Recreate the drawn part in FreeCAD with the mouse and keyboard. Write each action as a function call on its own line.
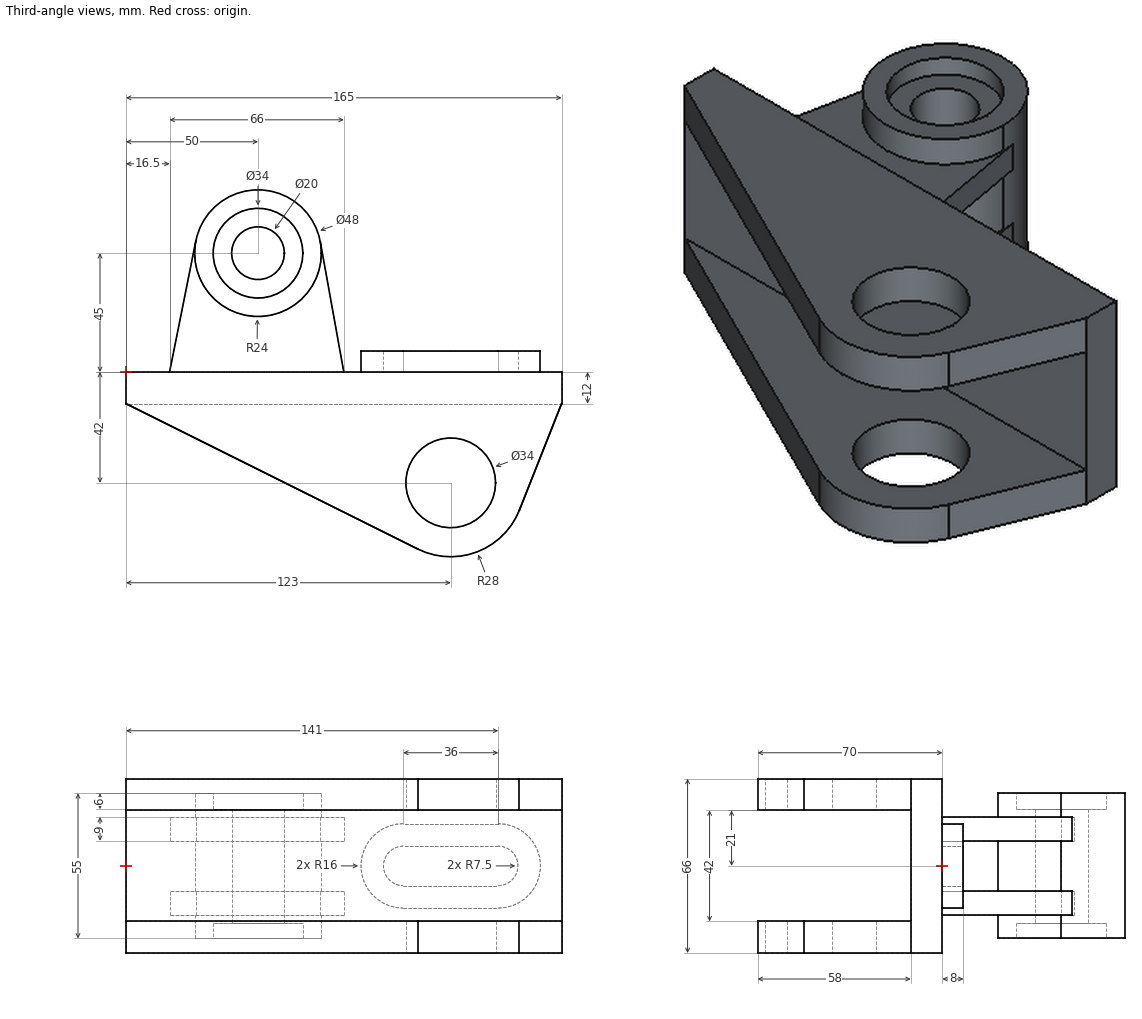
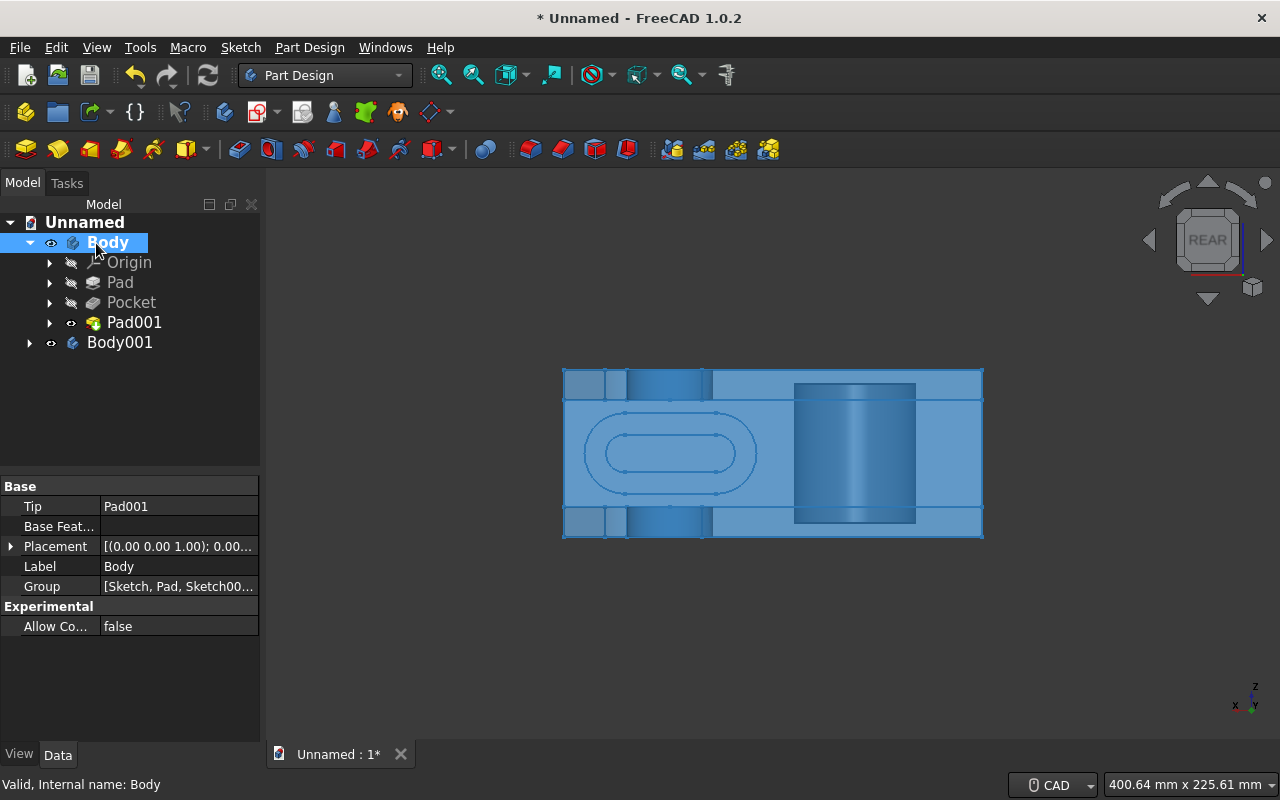
click(96, 243)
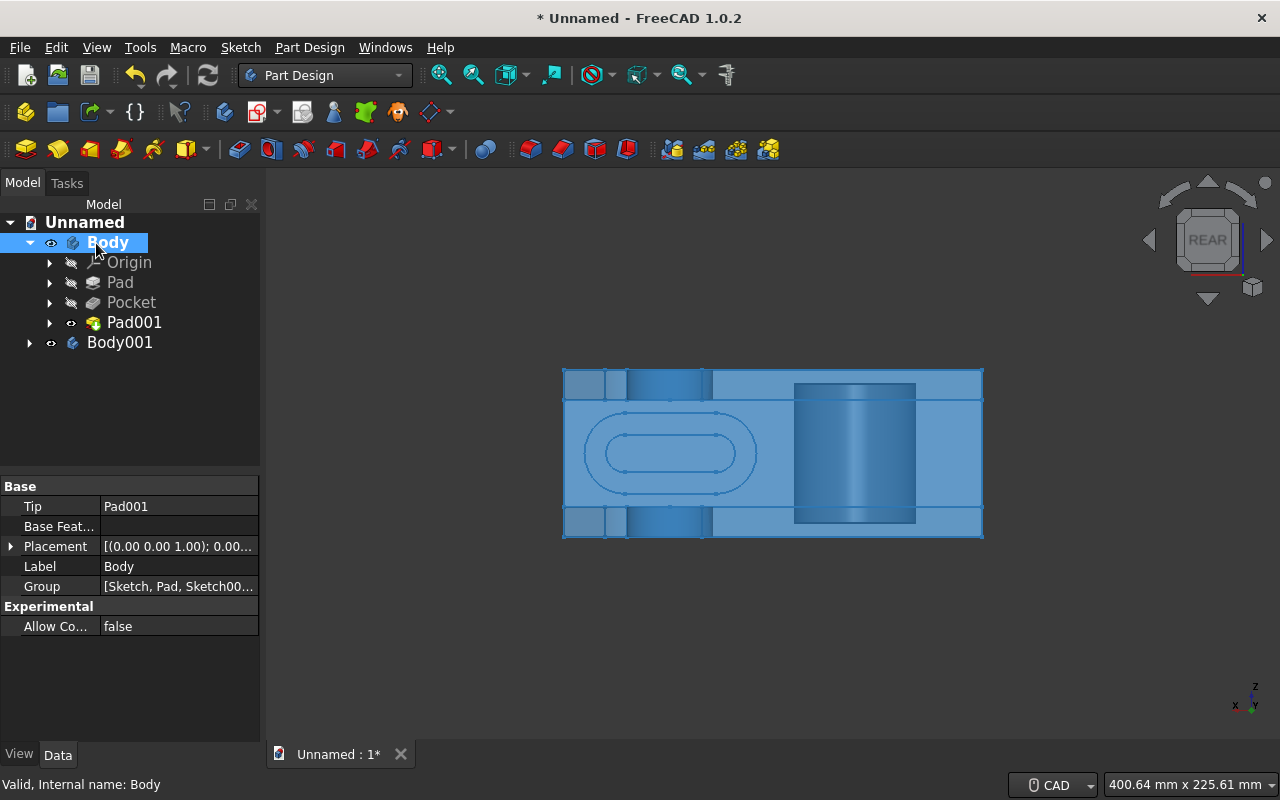
click(146, 626)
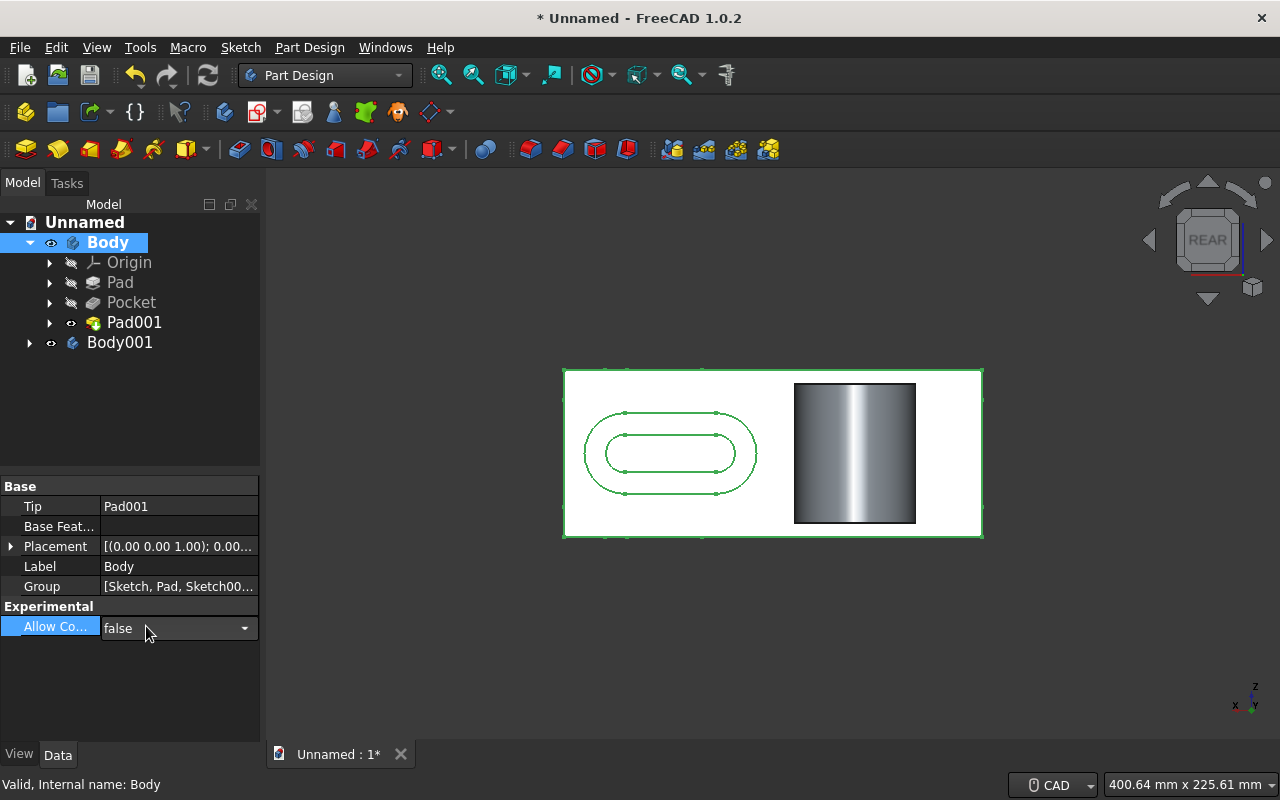
click(146, 626)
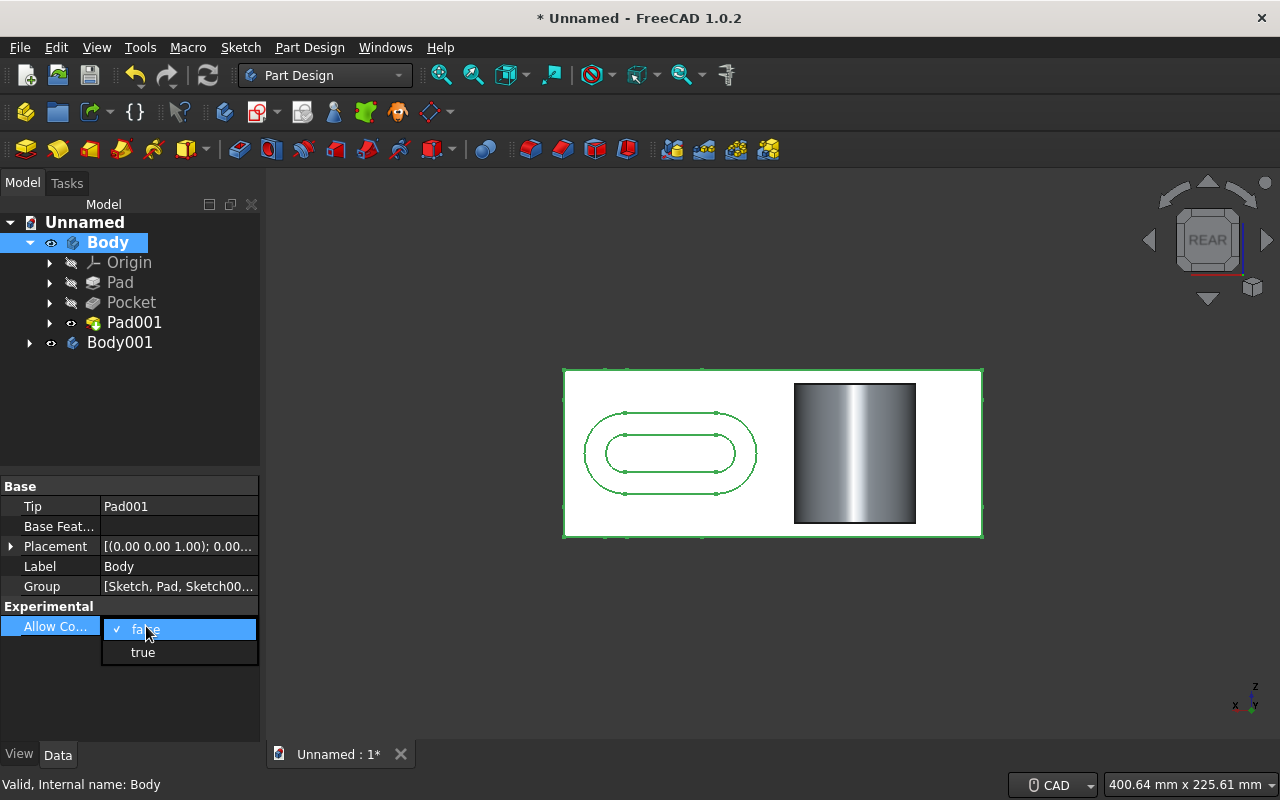
click(179, 652)
key(Return)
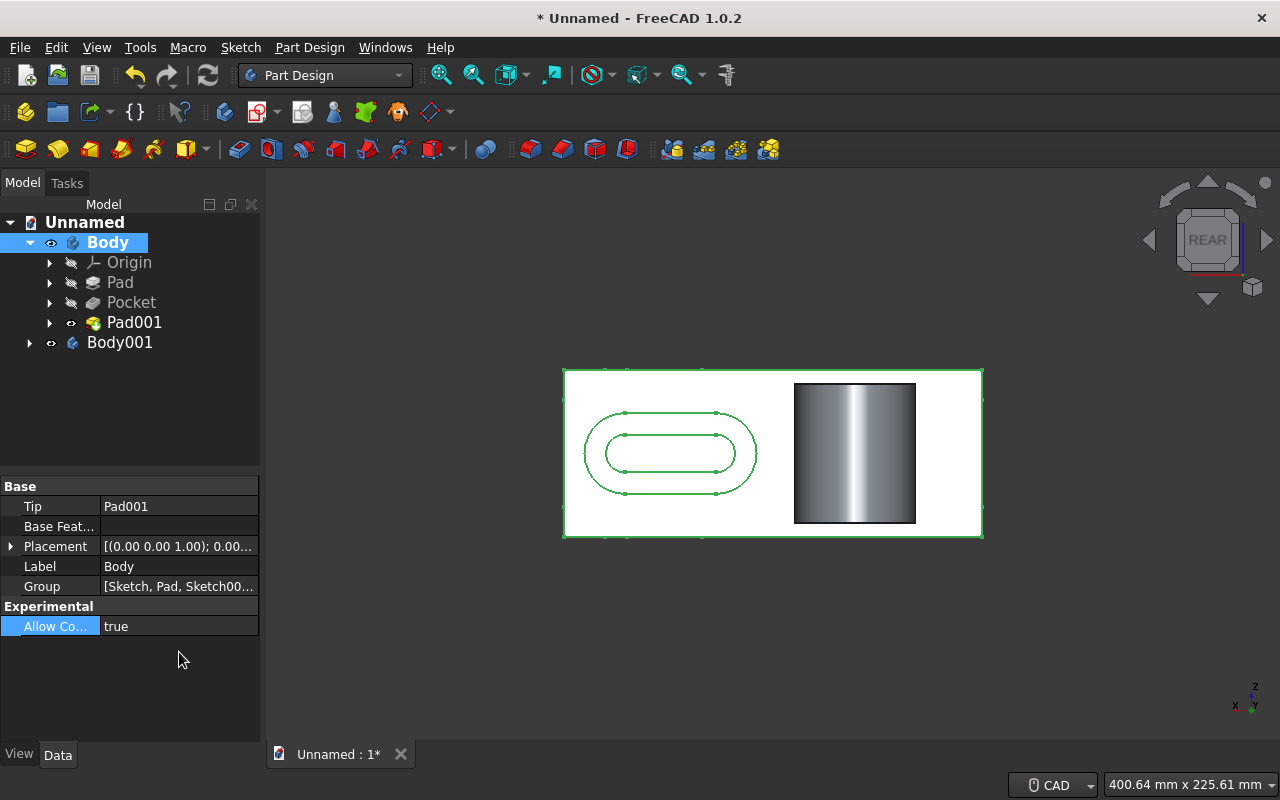
click(96, 343)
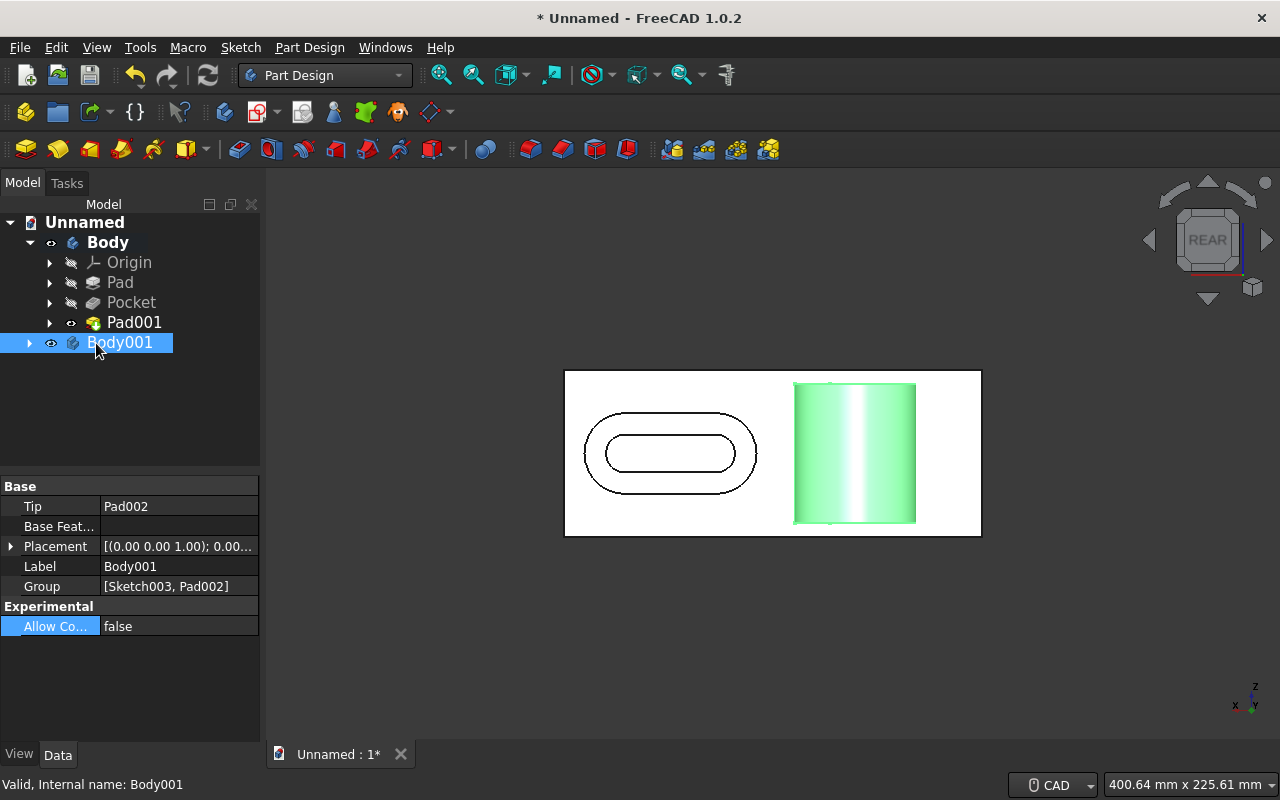
click(486, 150)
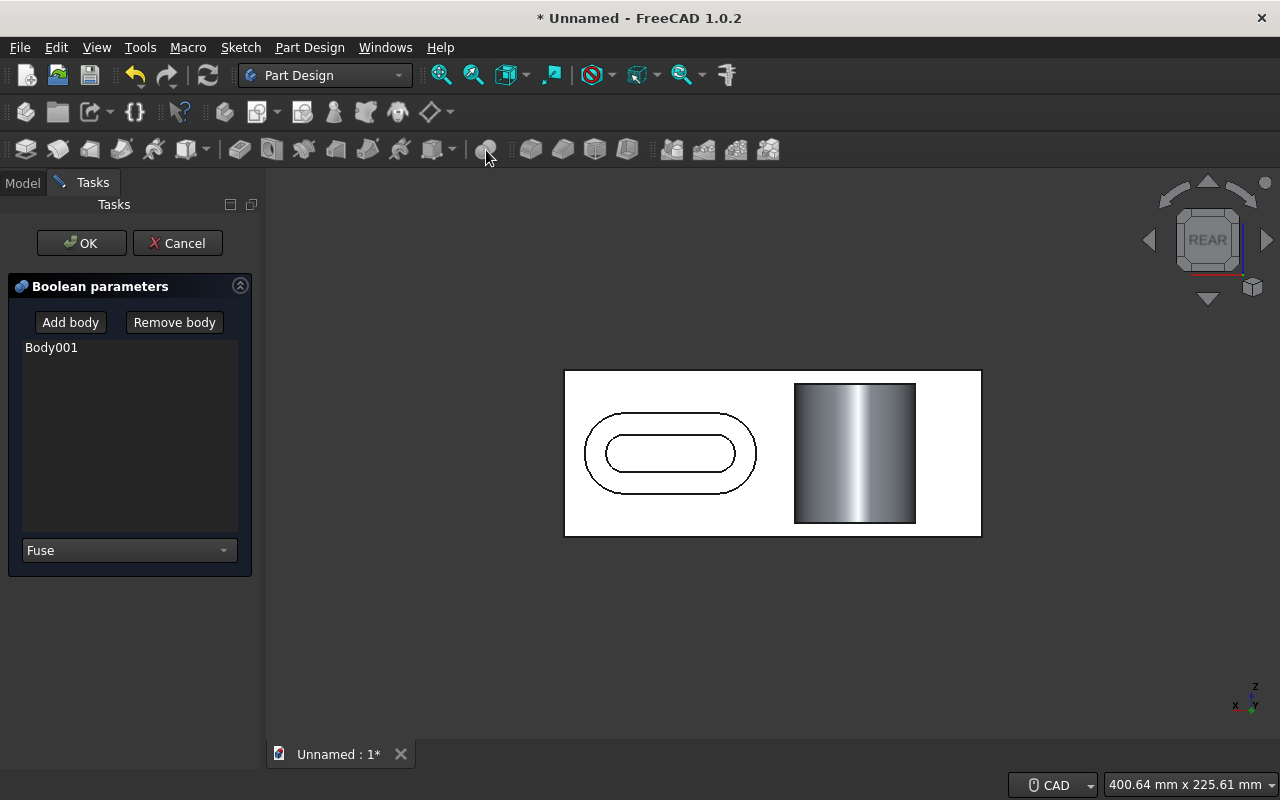
click(82, 243)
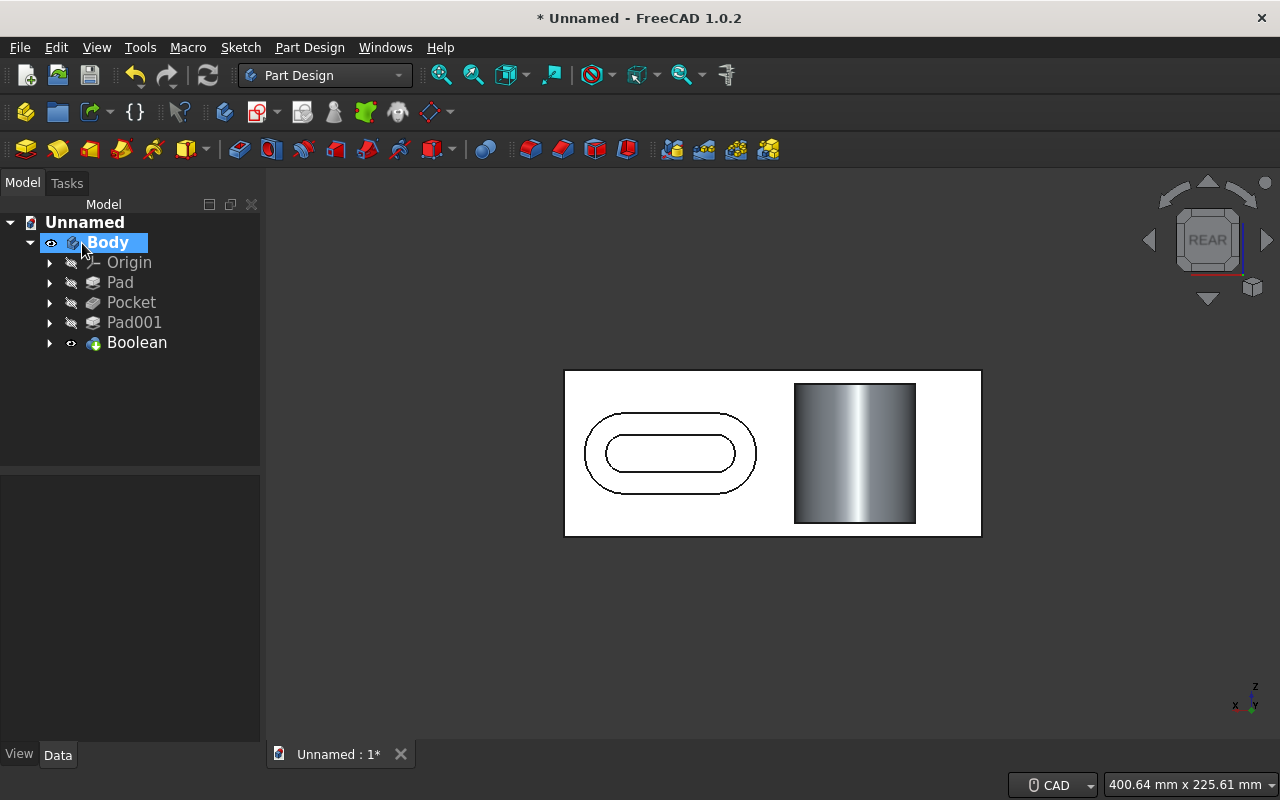
key(v)
key(f)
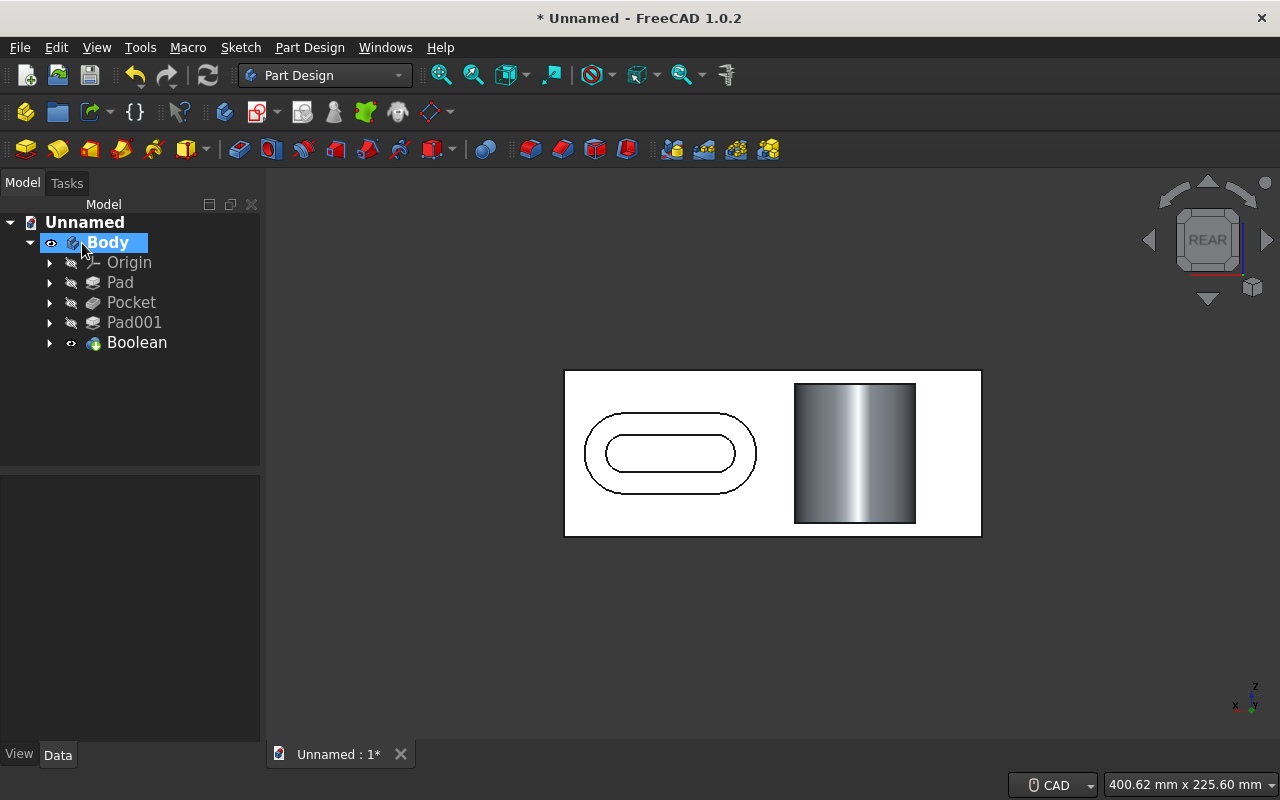
click(50, 263)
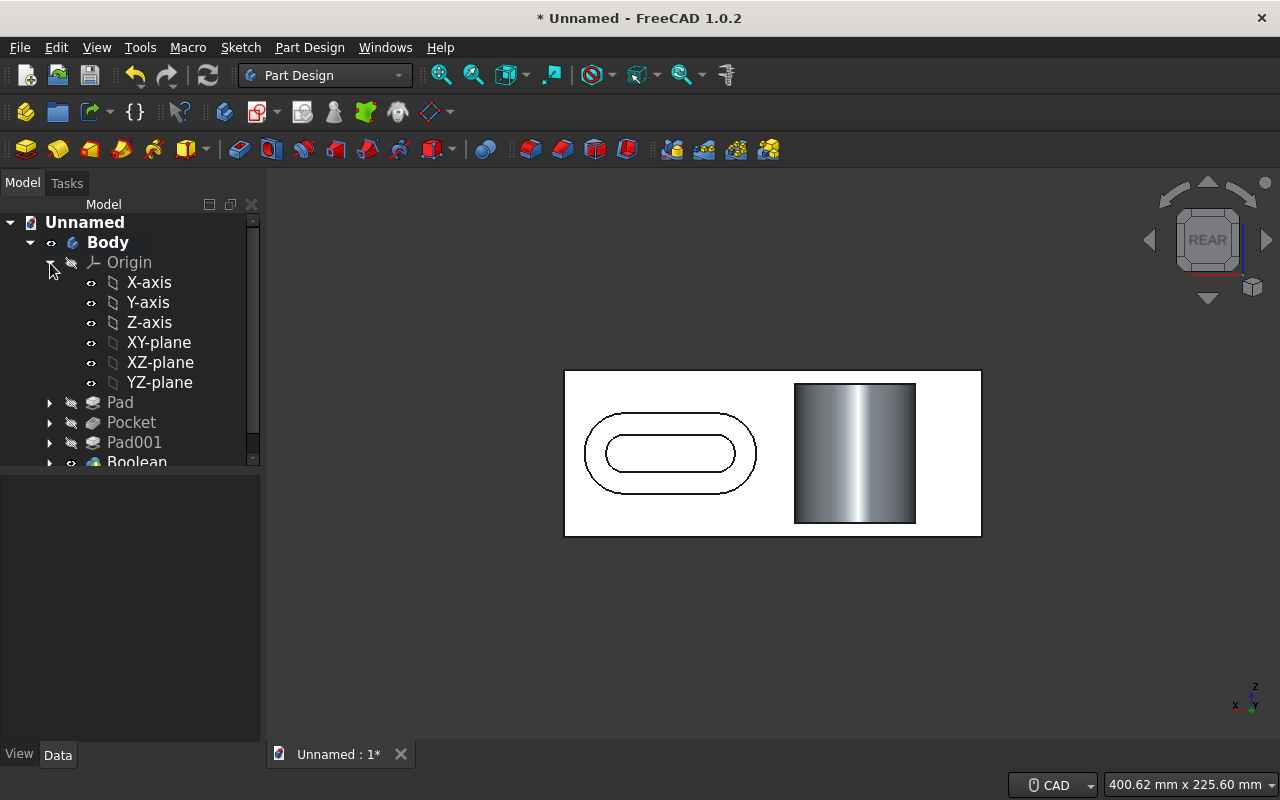
click(136, 343)